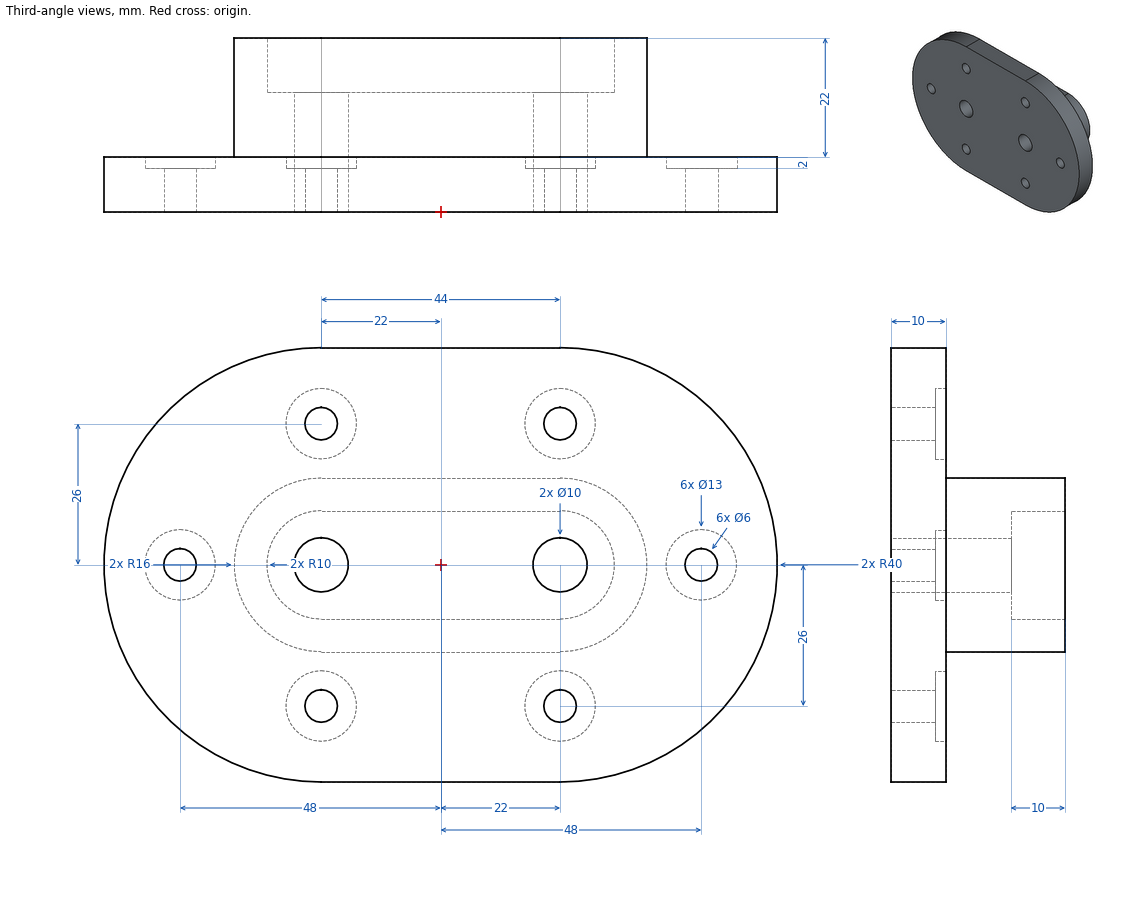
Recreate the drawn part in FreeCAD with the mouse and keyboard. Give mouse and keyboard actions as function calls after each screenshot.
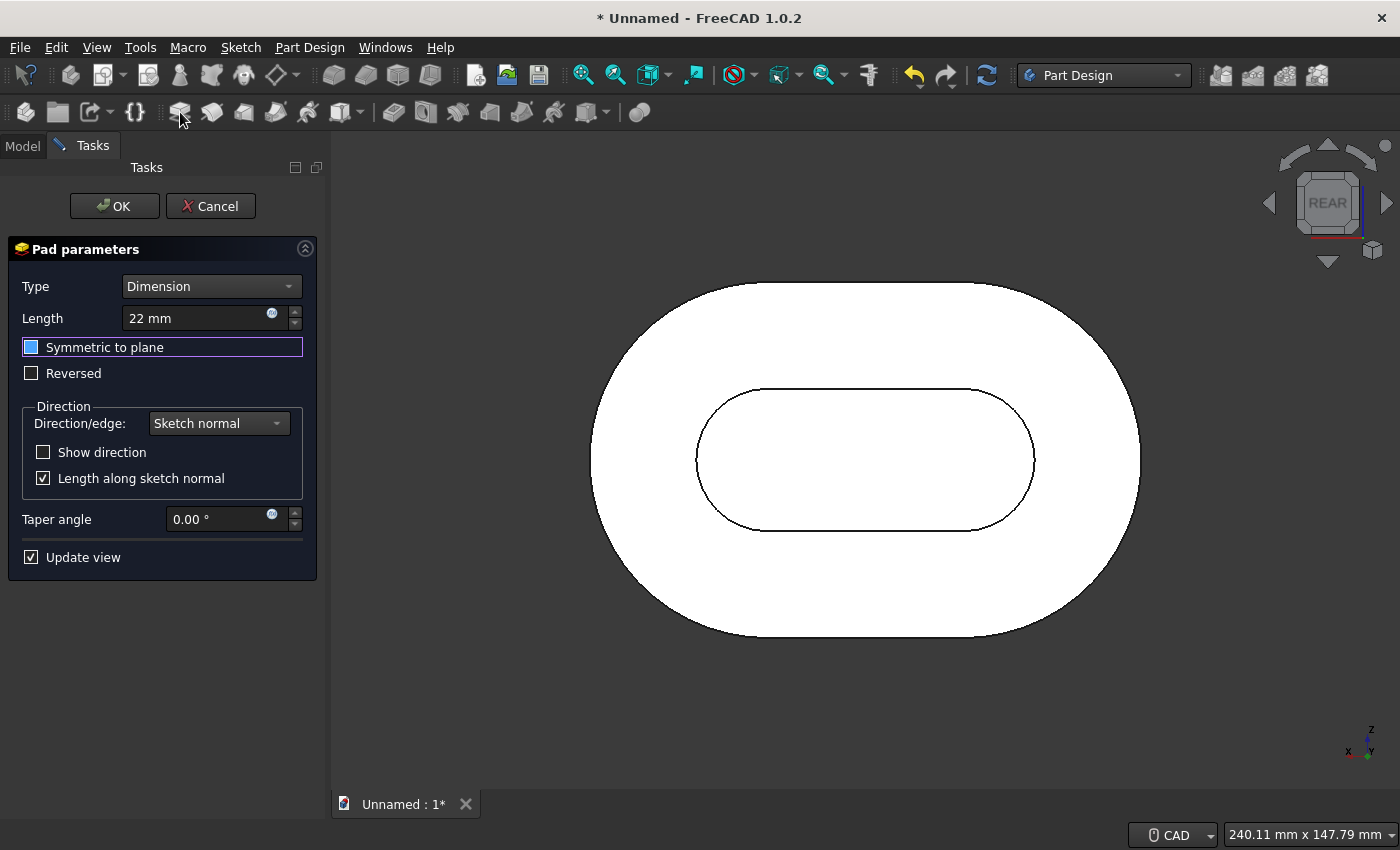
click(115, 206)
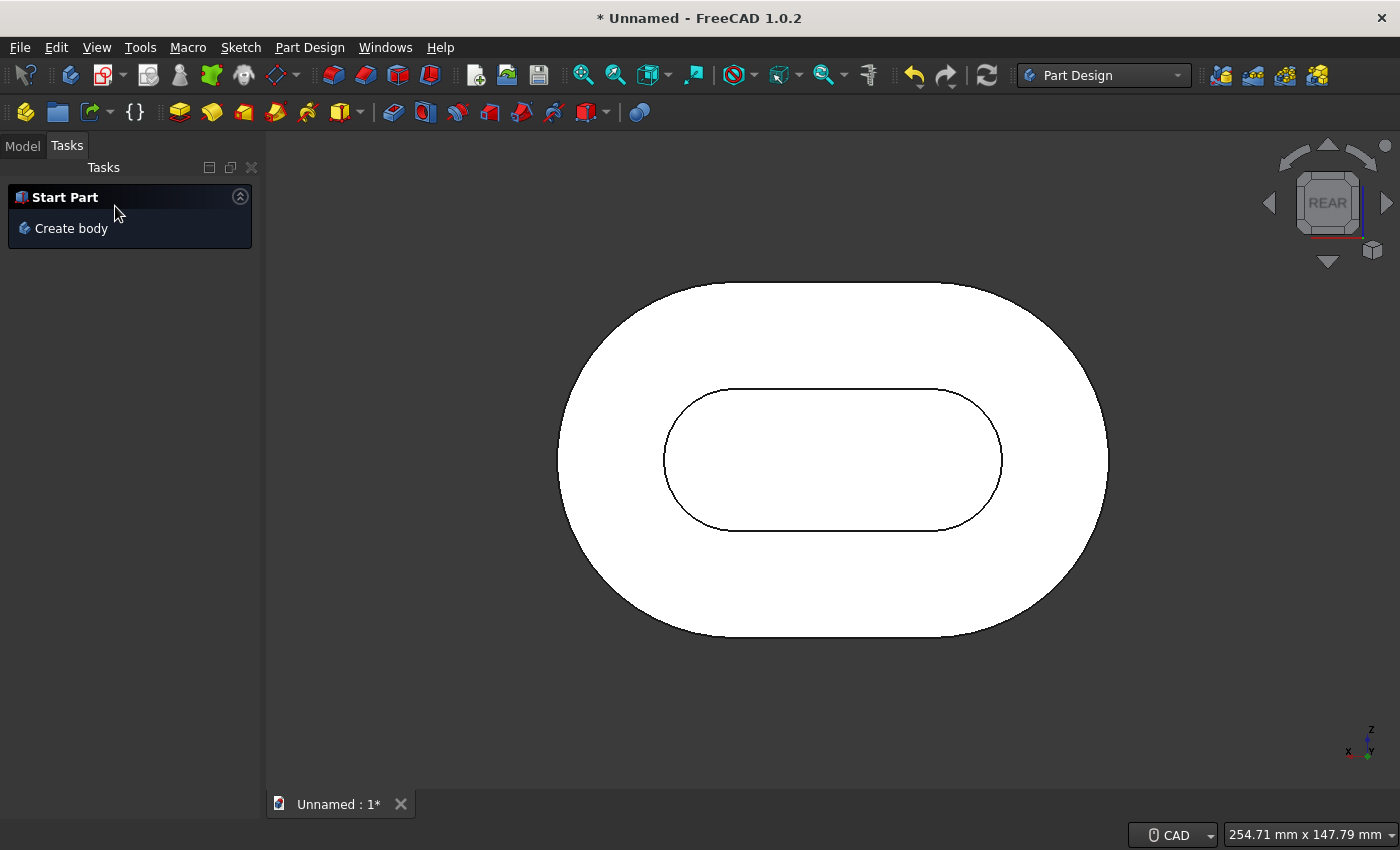
click(881, 459)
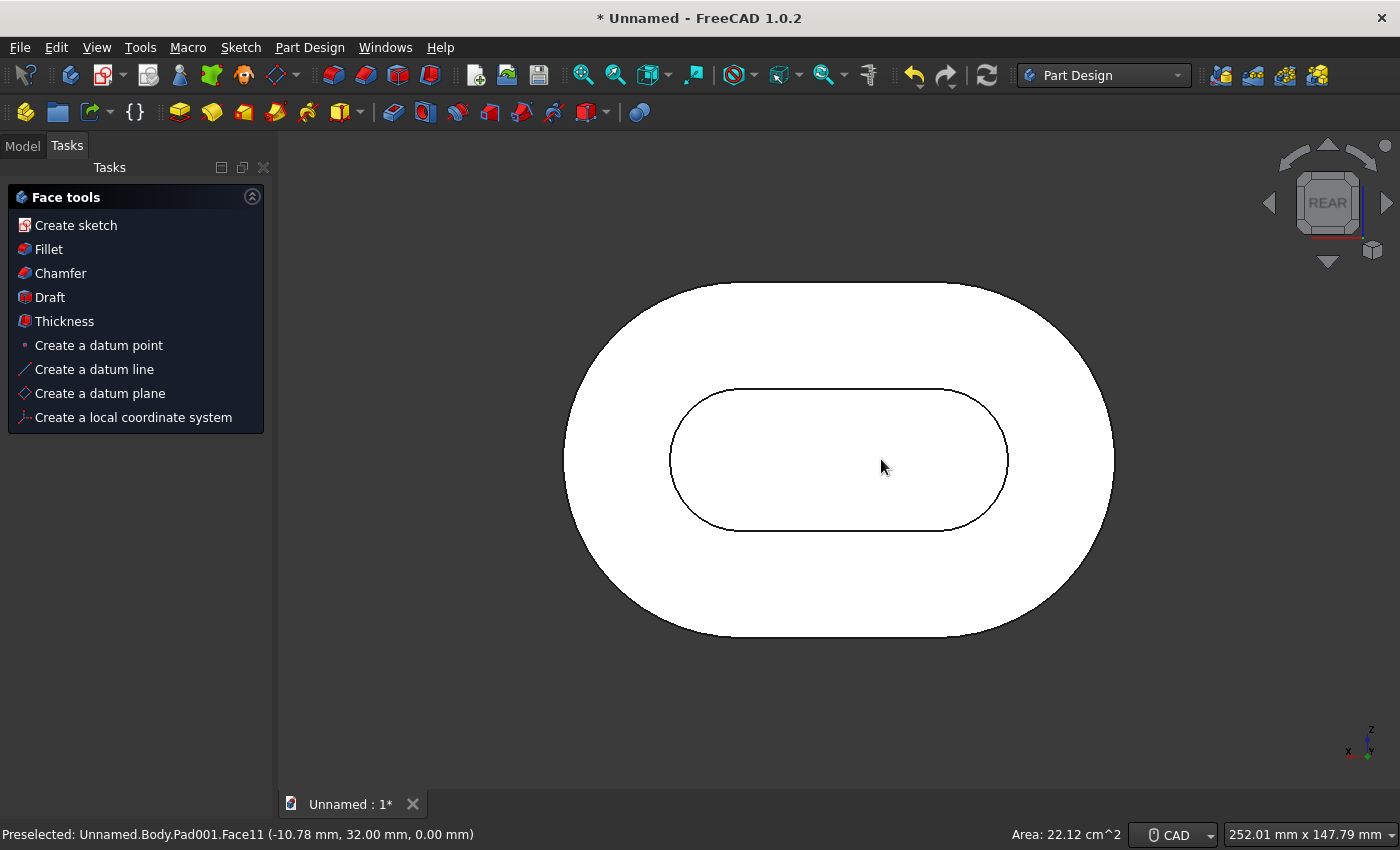
click(104, 76)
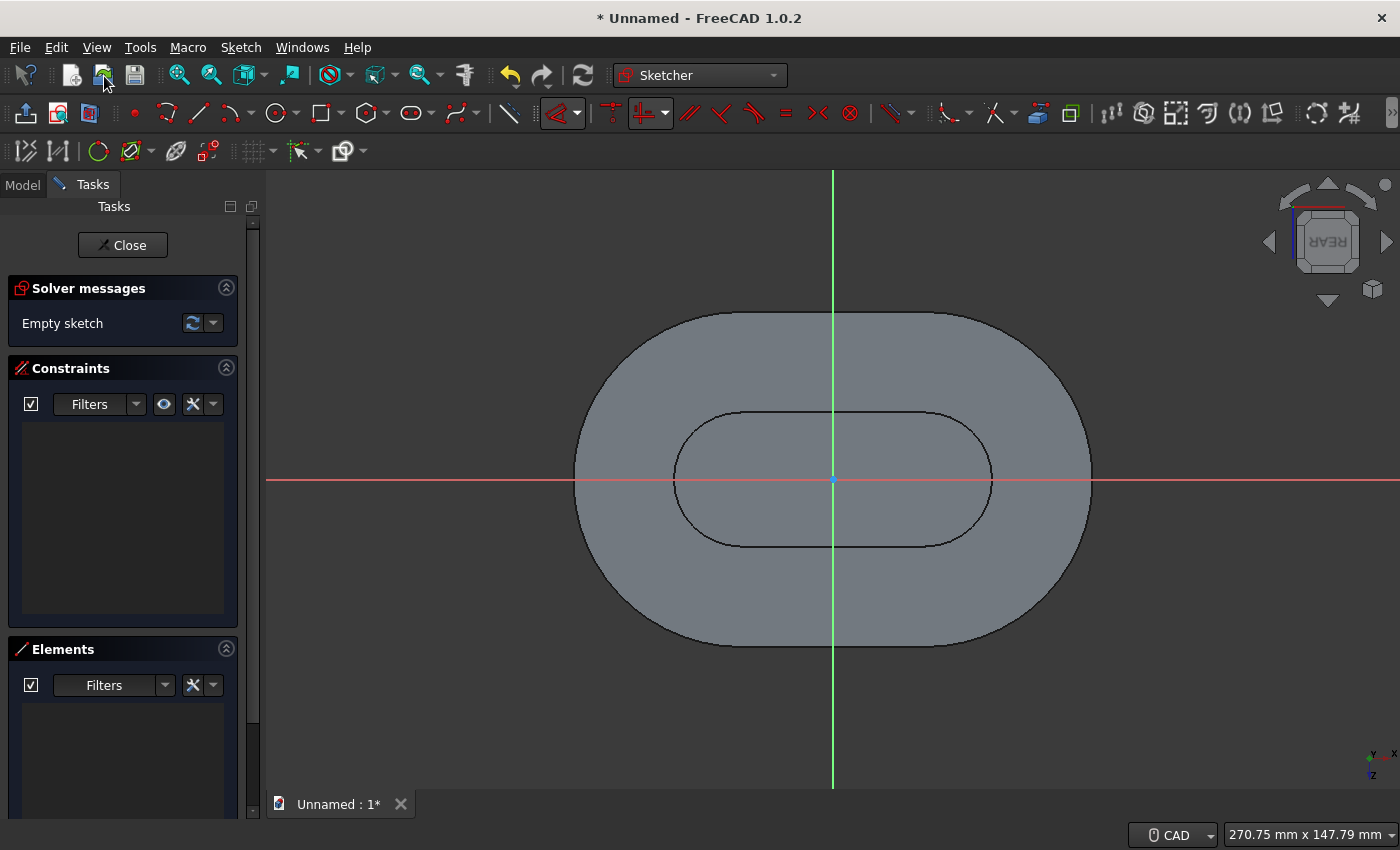
scroll(873, 479, up, 5)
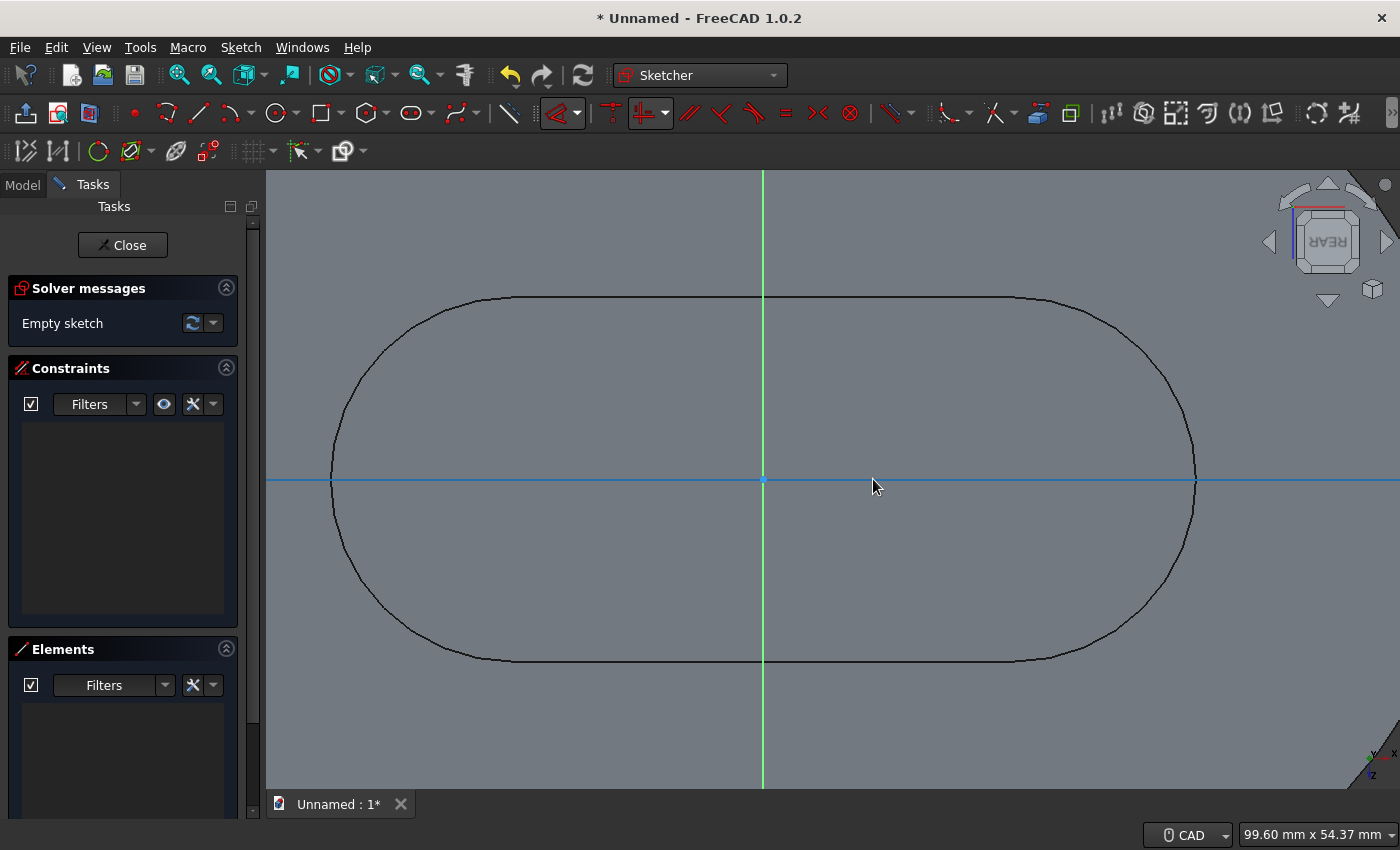
key(g)
key(s)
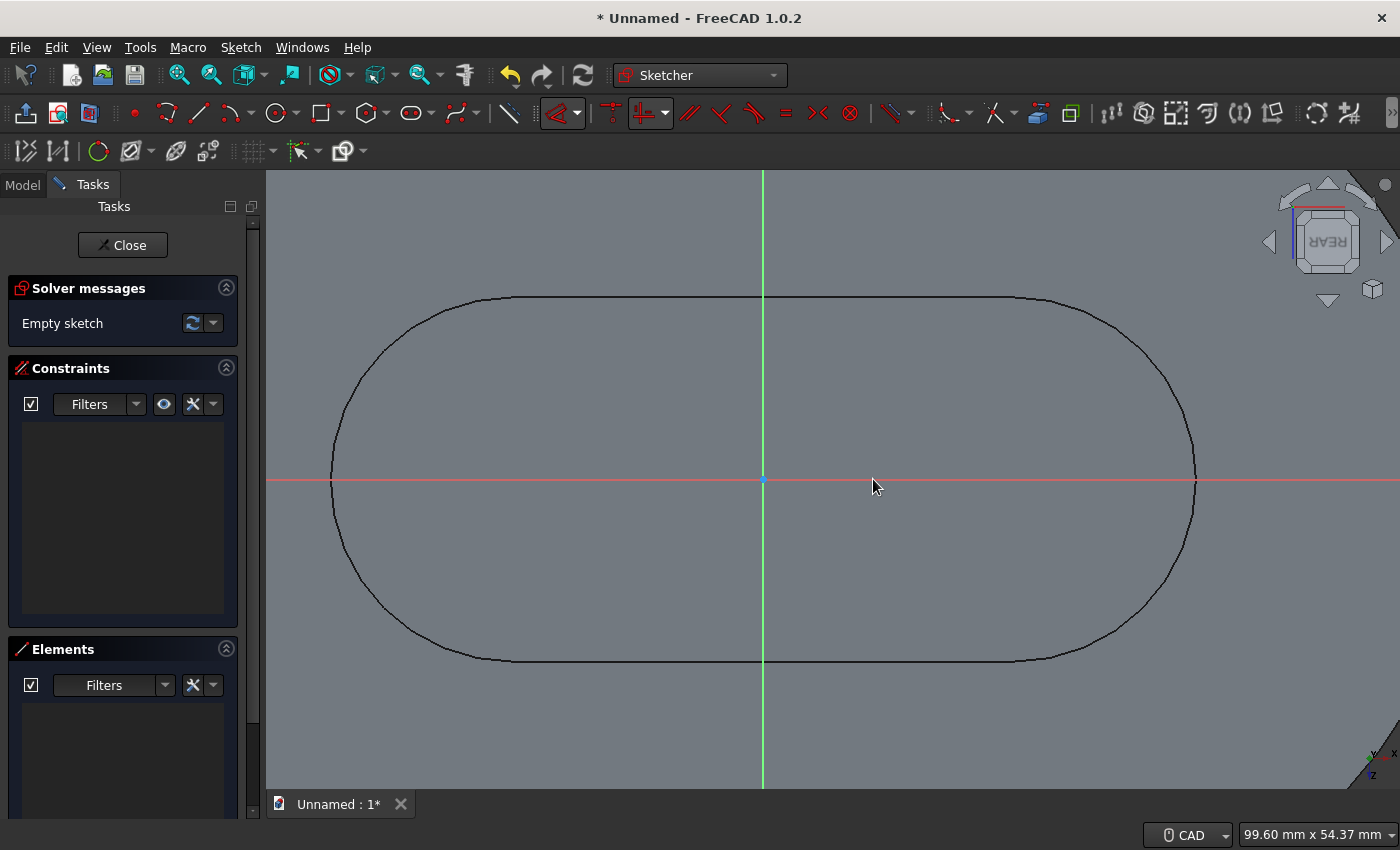
click(513, 479)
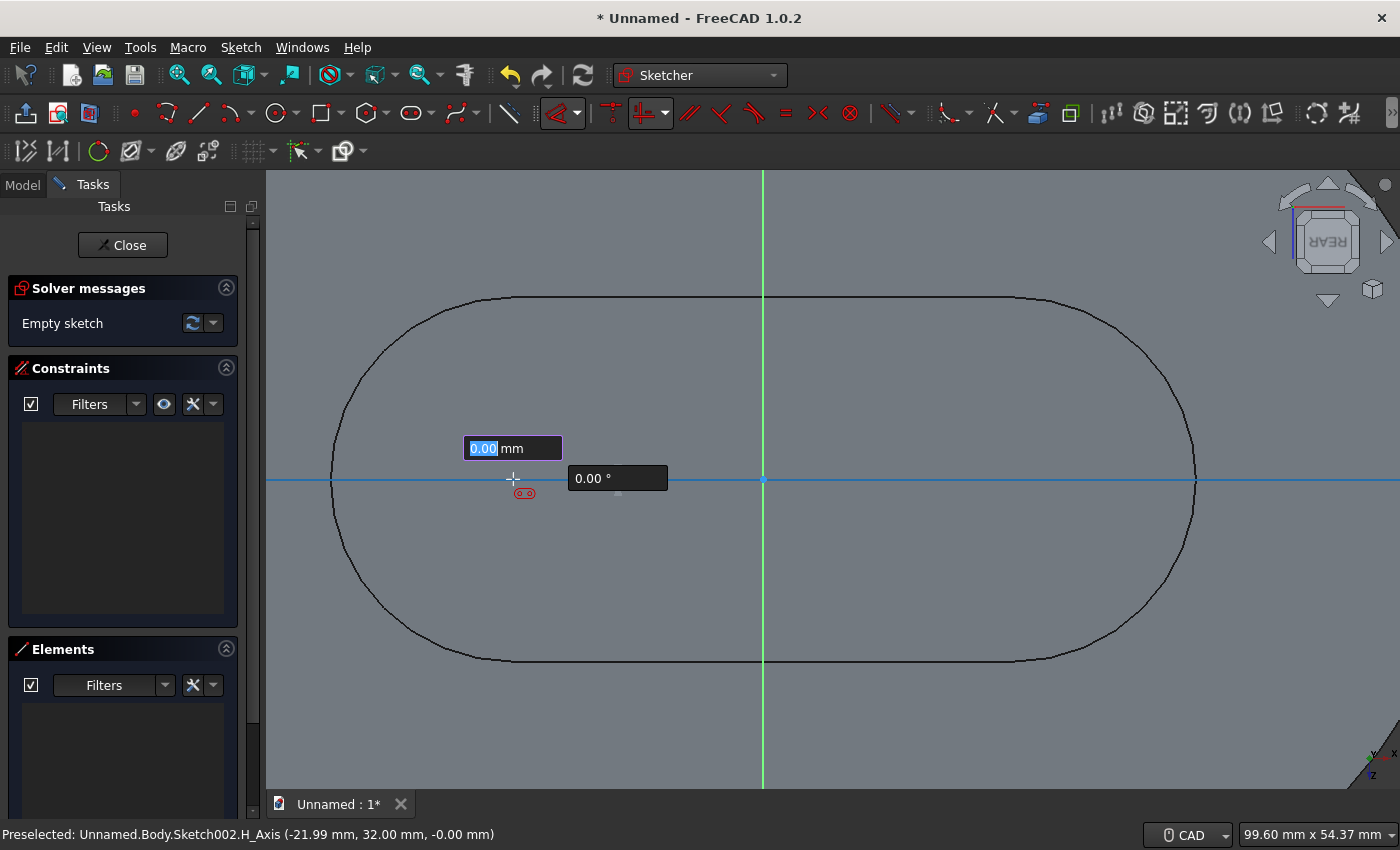
click(1014, 470)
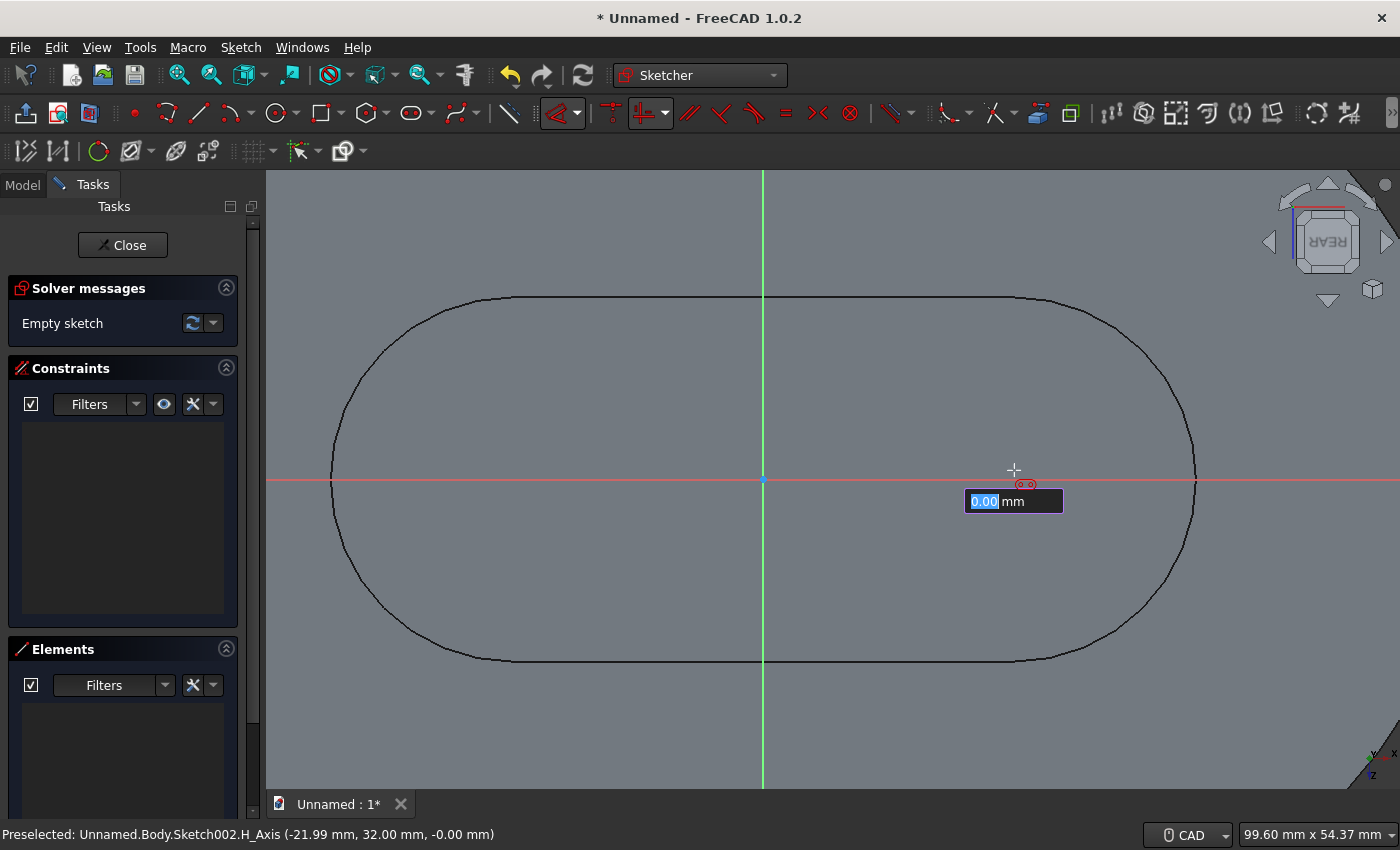
click(838, 366)
key(Escape)